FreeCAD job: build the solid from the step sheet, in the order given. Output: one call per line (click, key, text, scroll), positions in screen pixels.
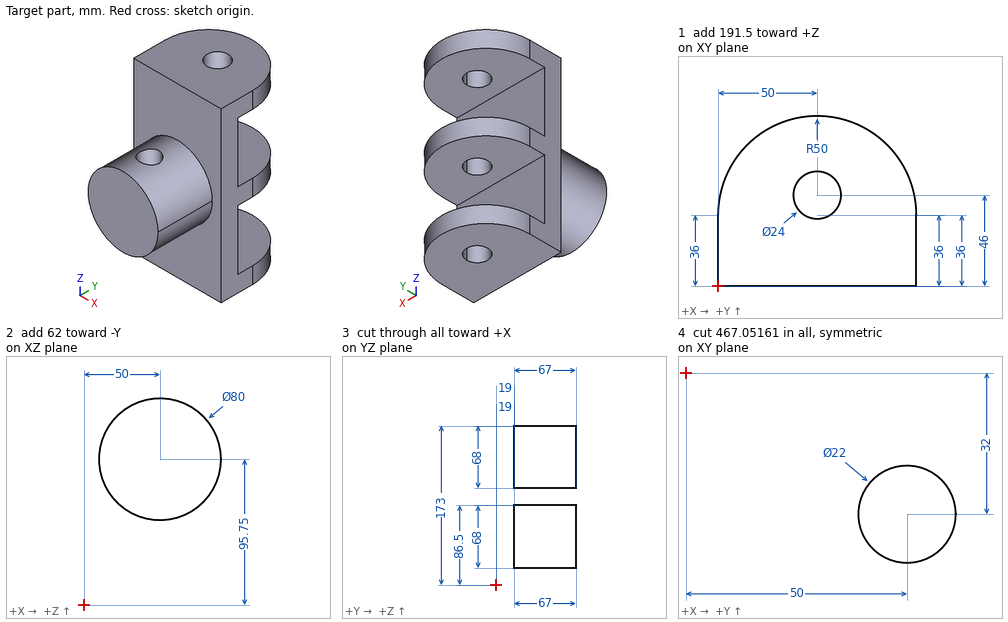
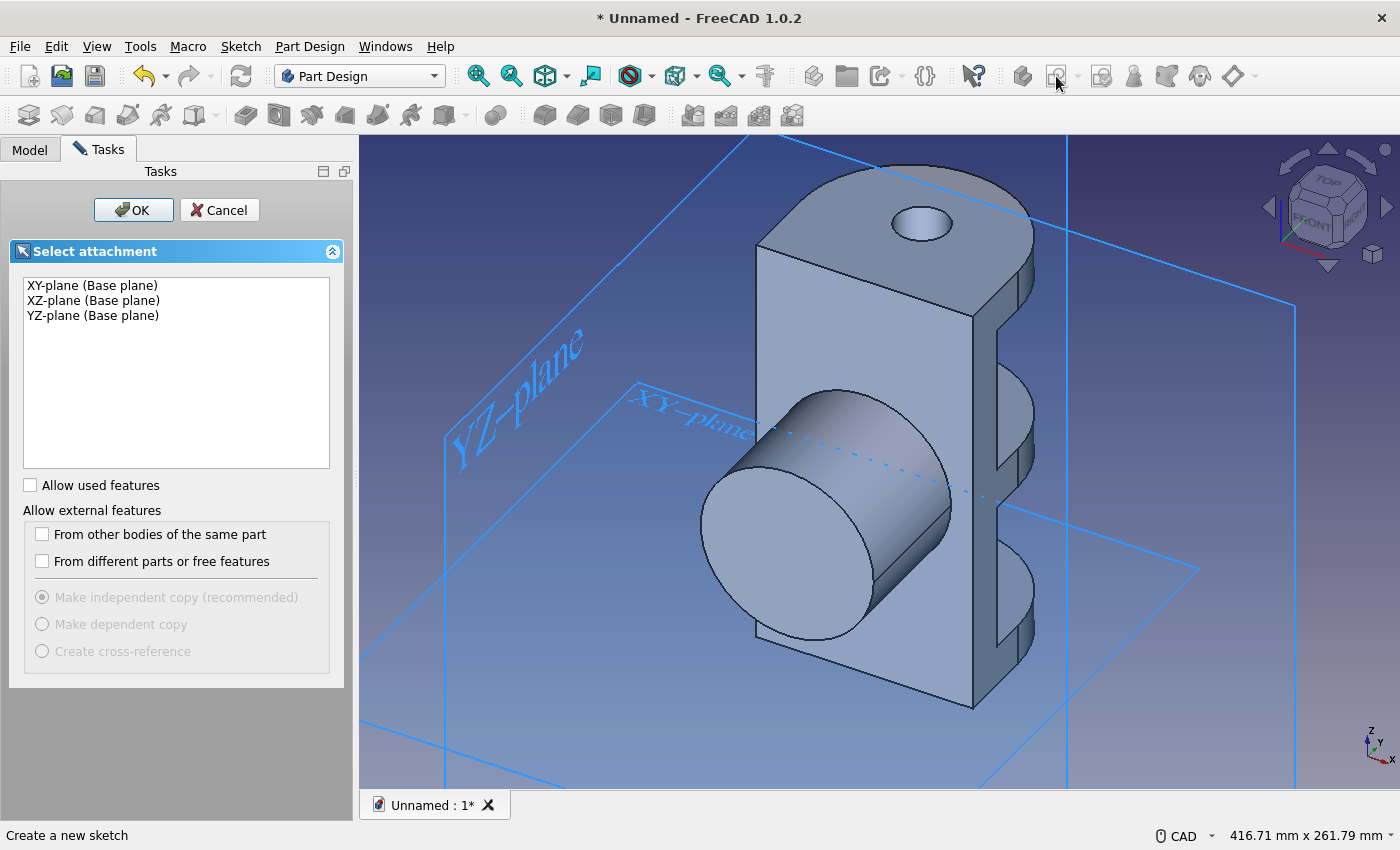
click(84, 286)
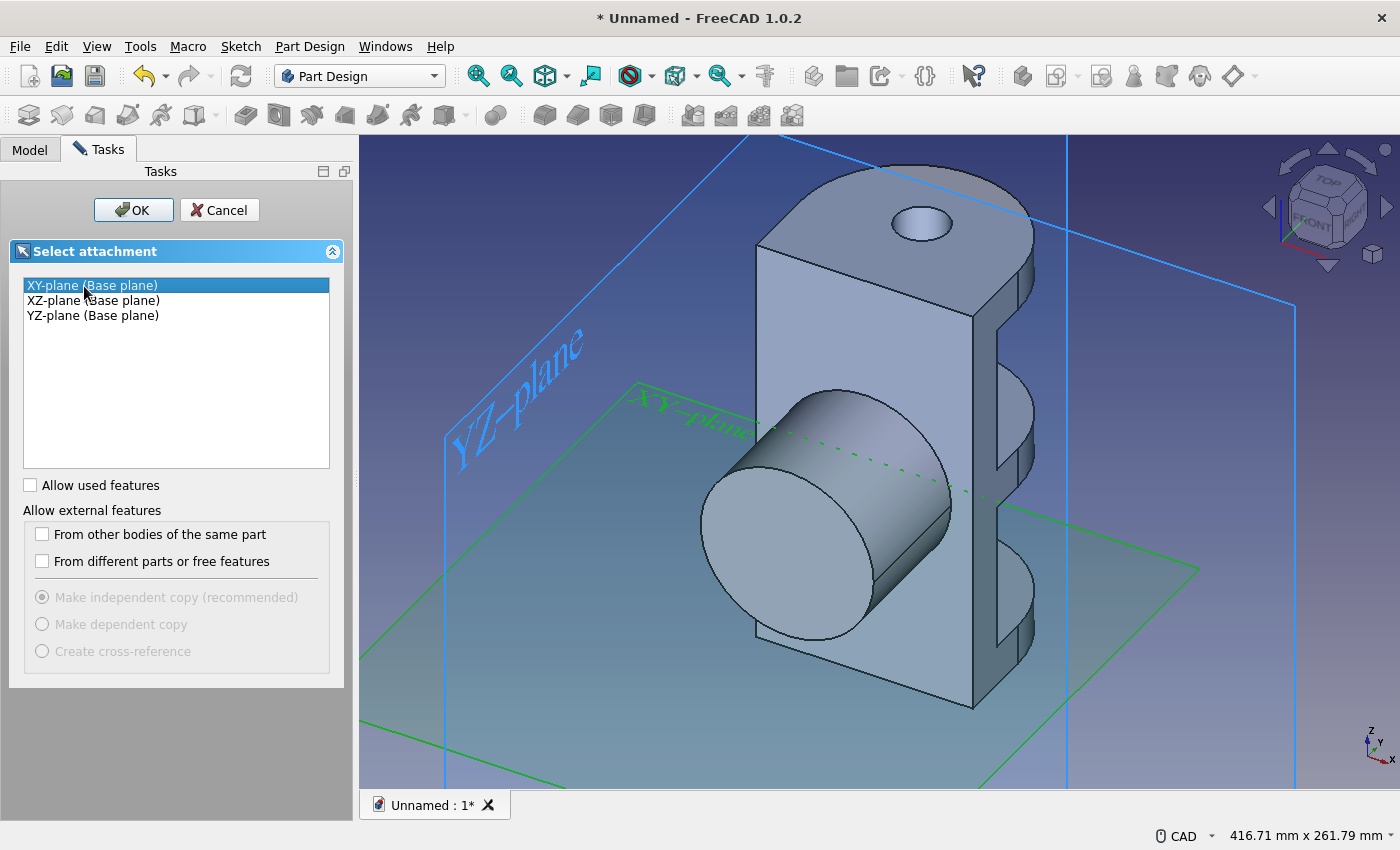
click(134, 210)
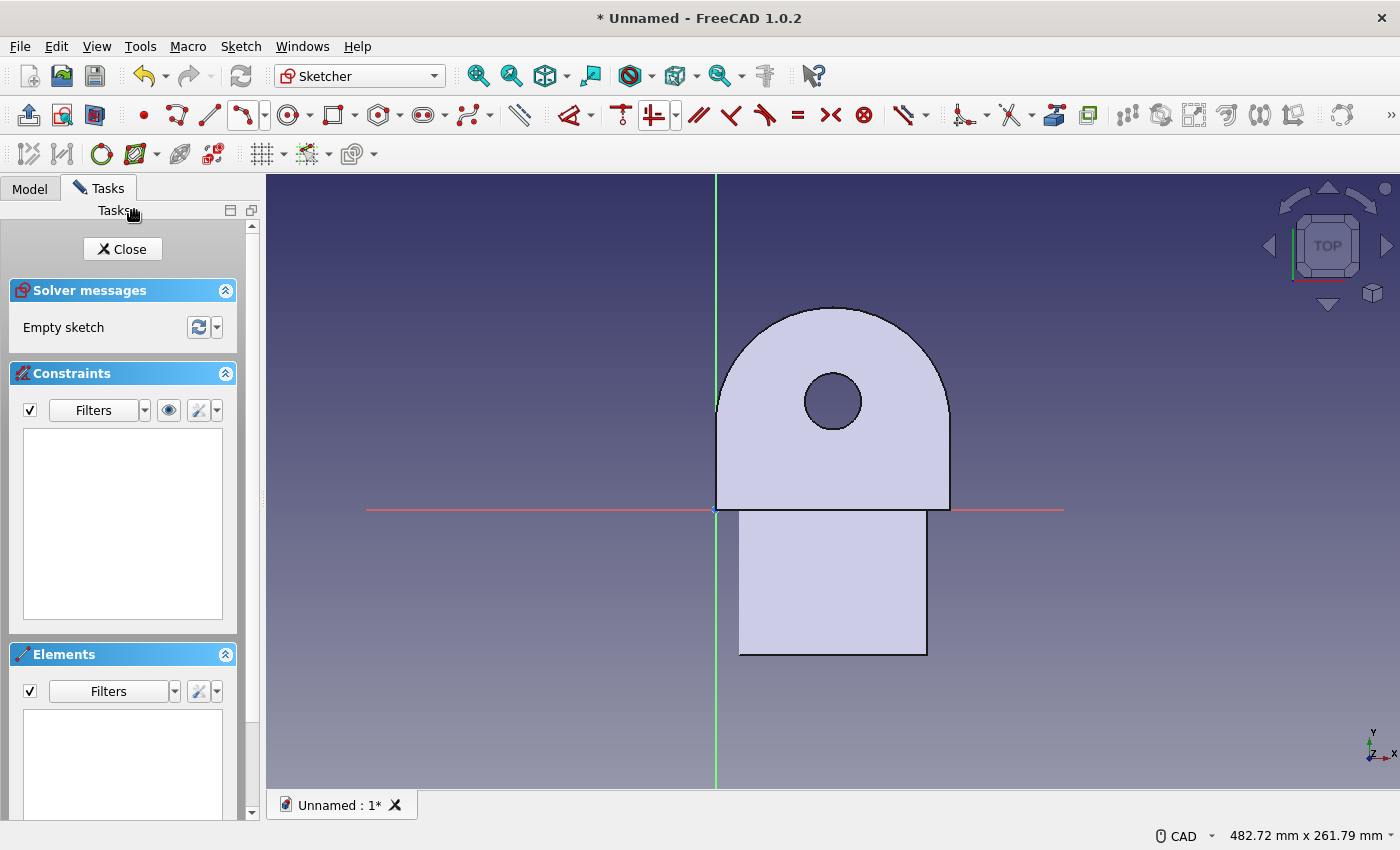
click(95, 116)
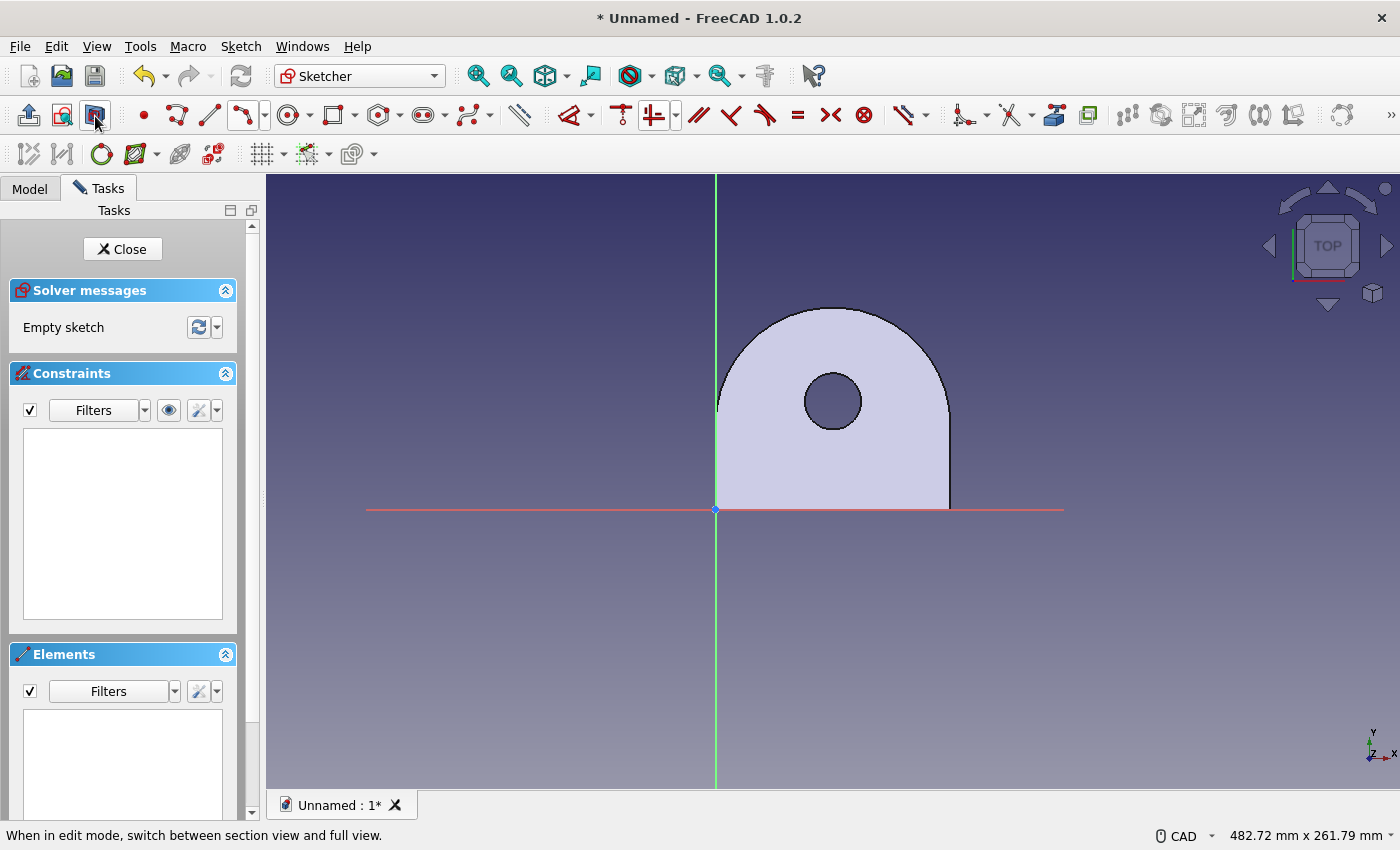
scroll(844, 601, up, 10)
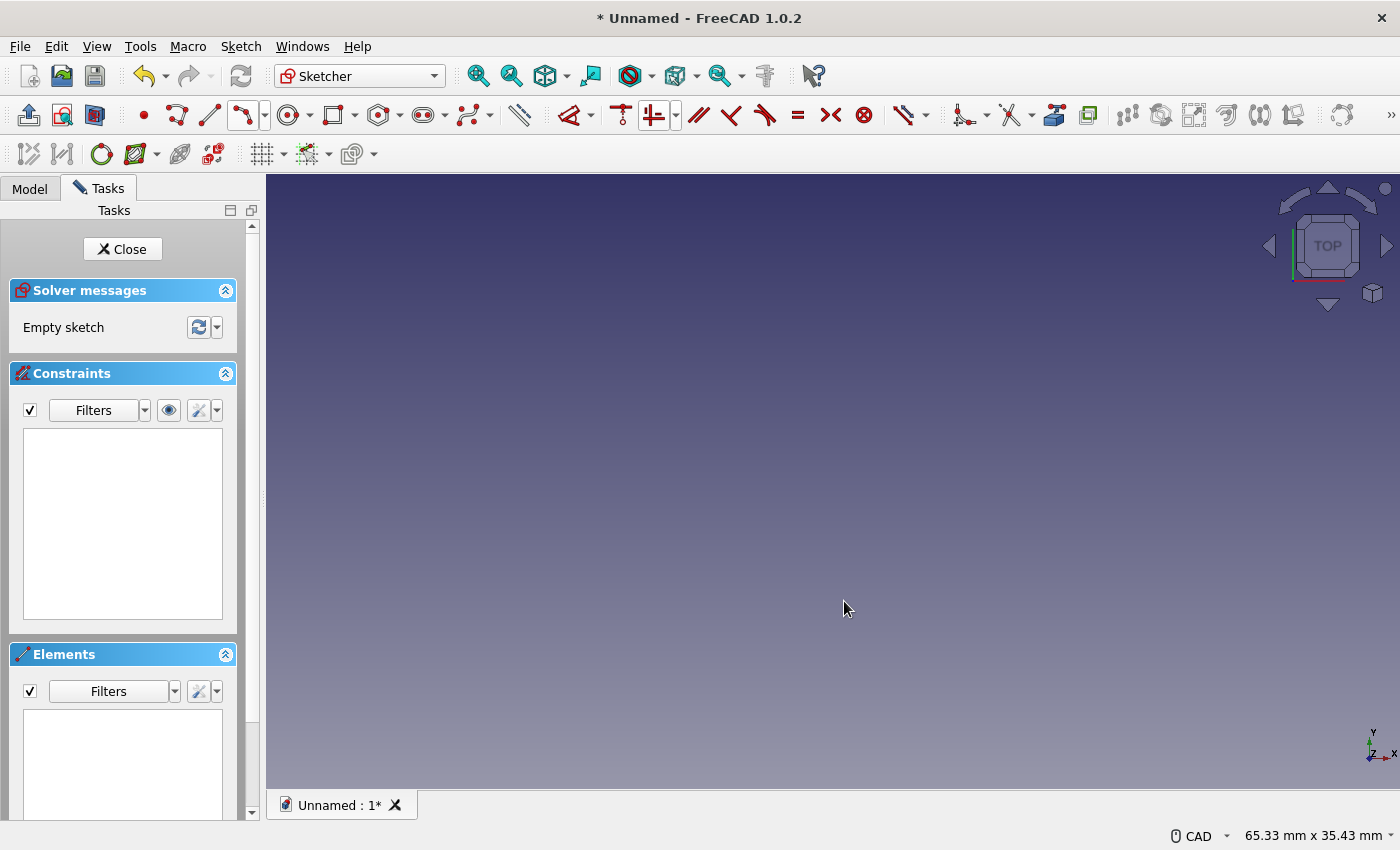
click(288, 116)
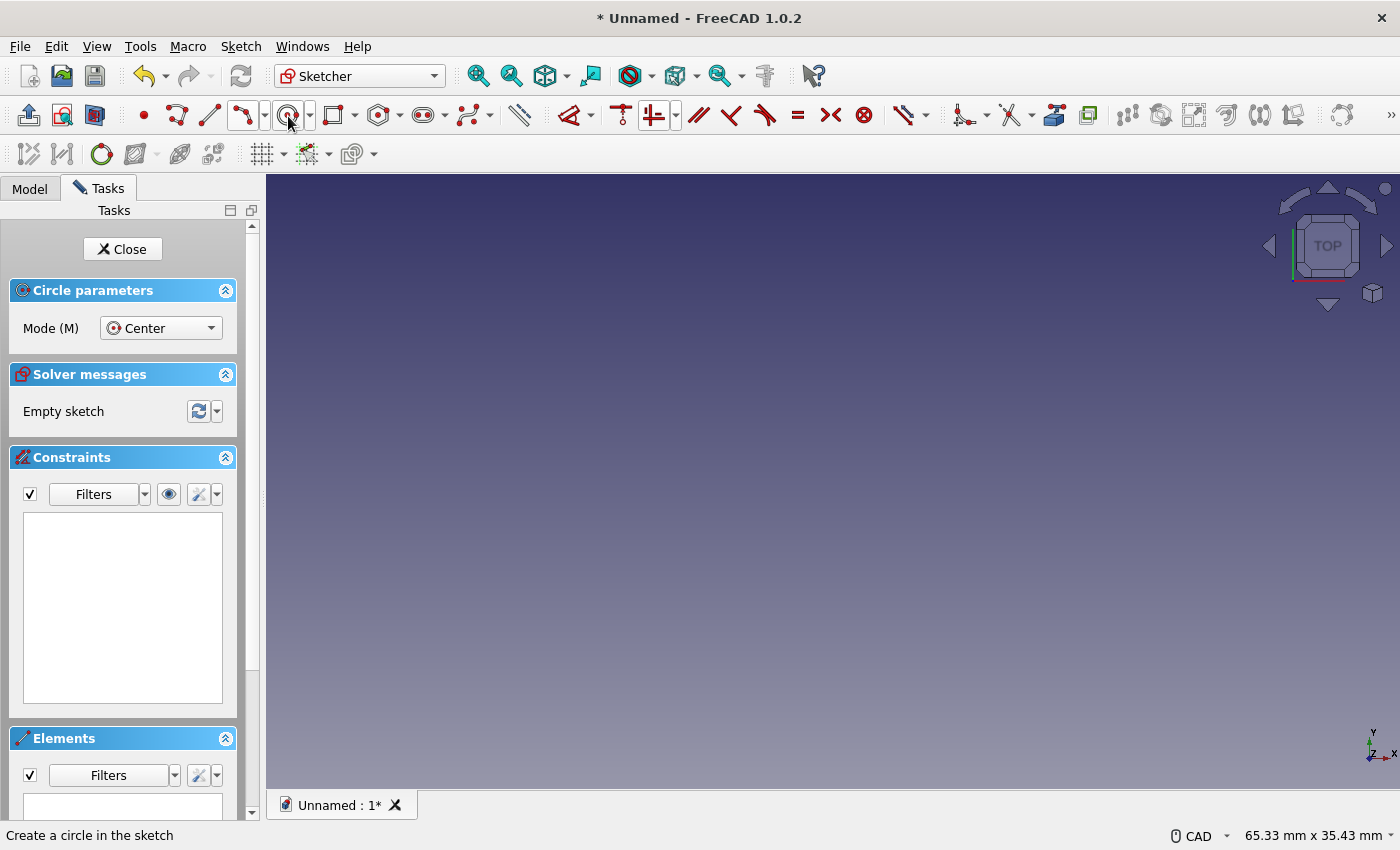
click(759, 476)
click(894, 341)
key(Escape)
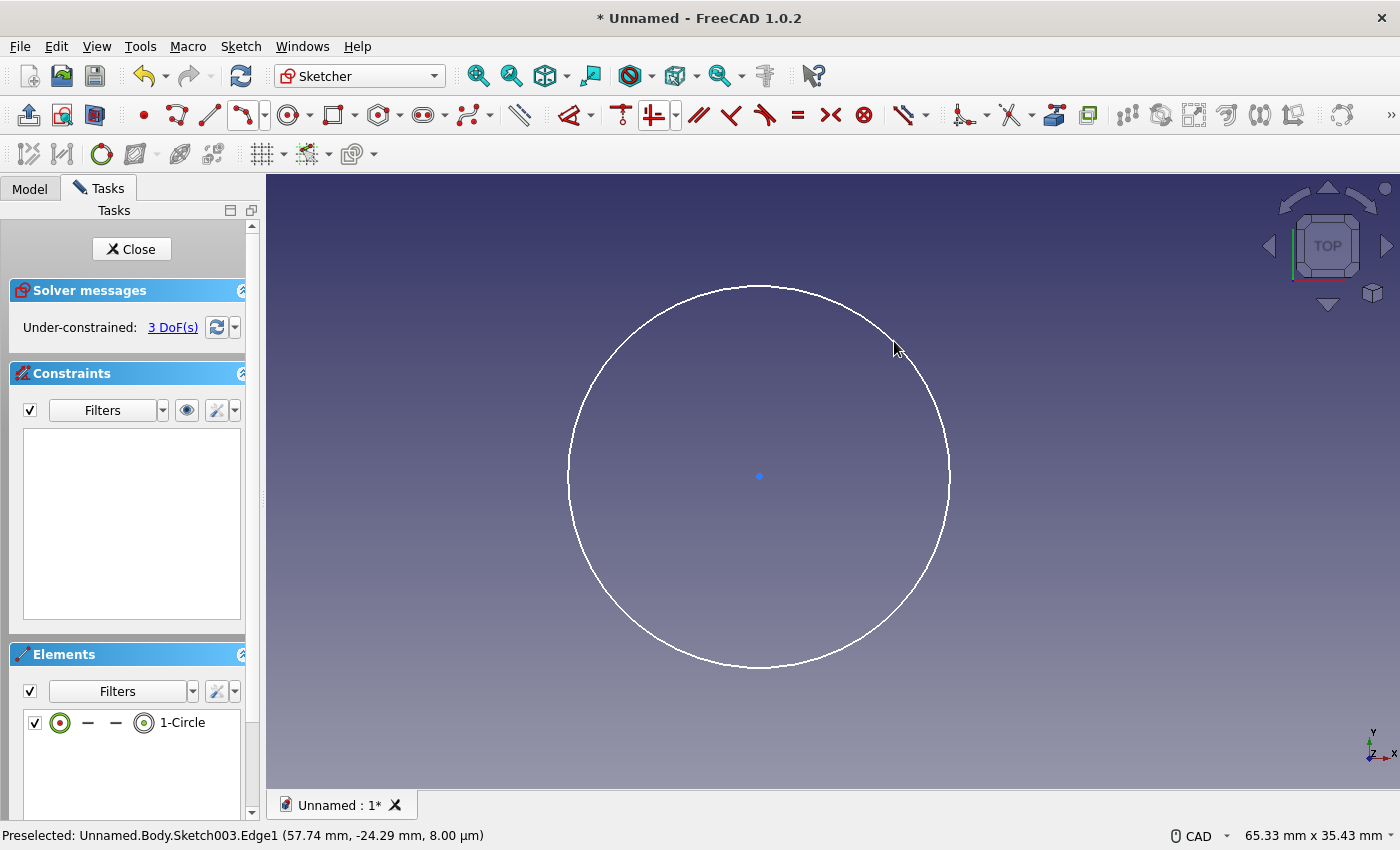
click(568, 116)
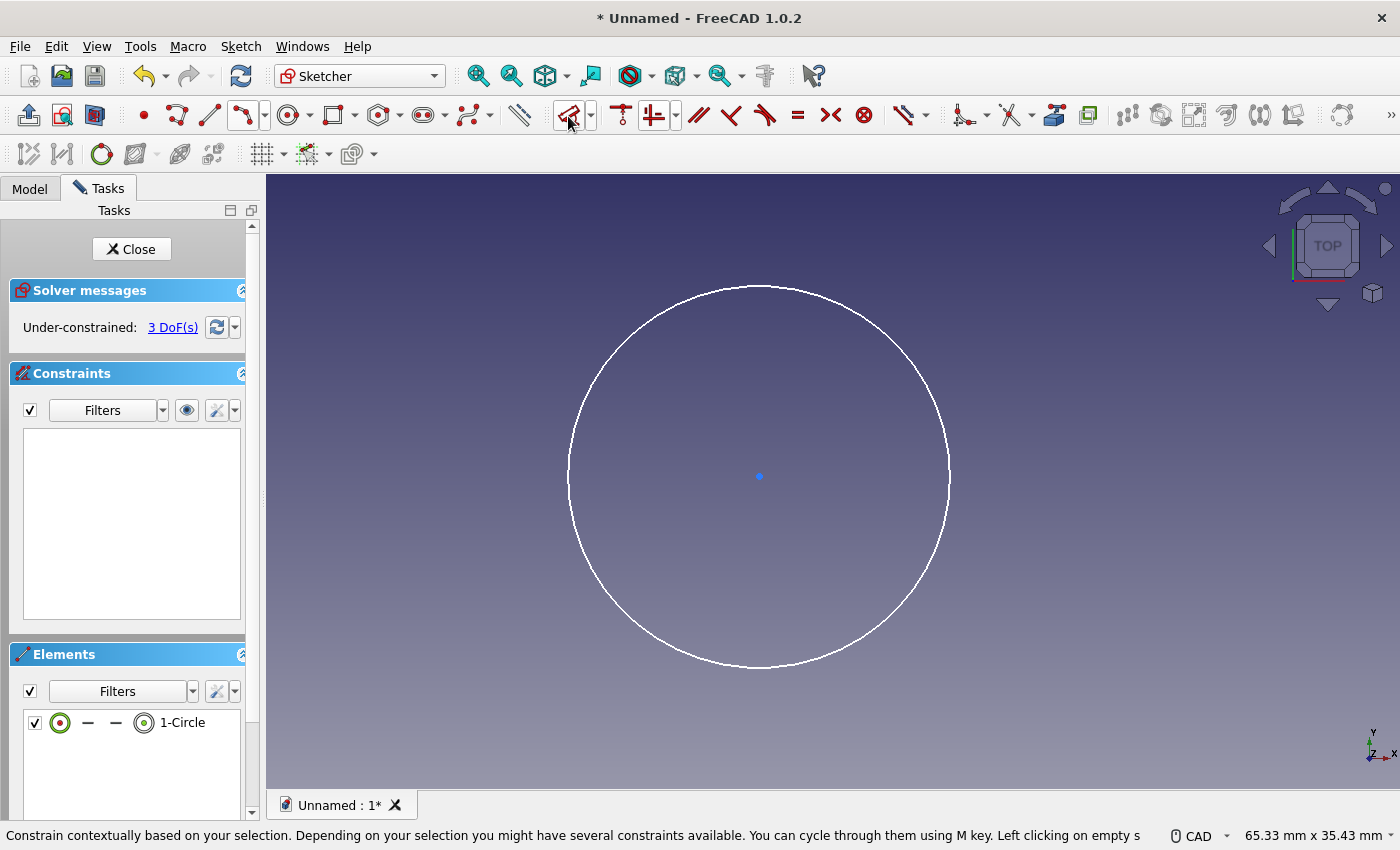
click(894, 342)
click(917, 319)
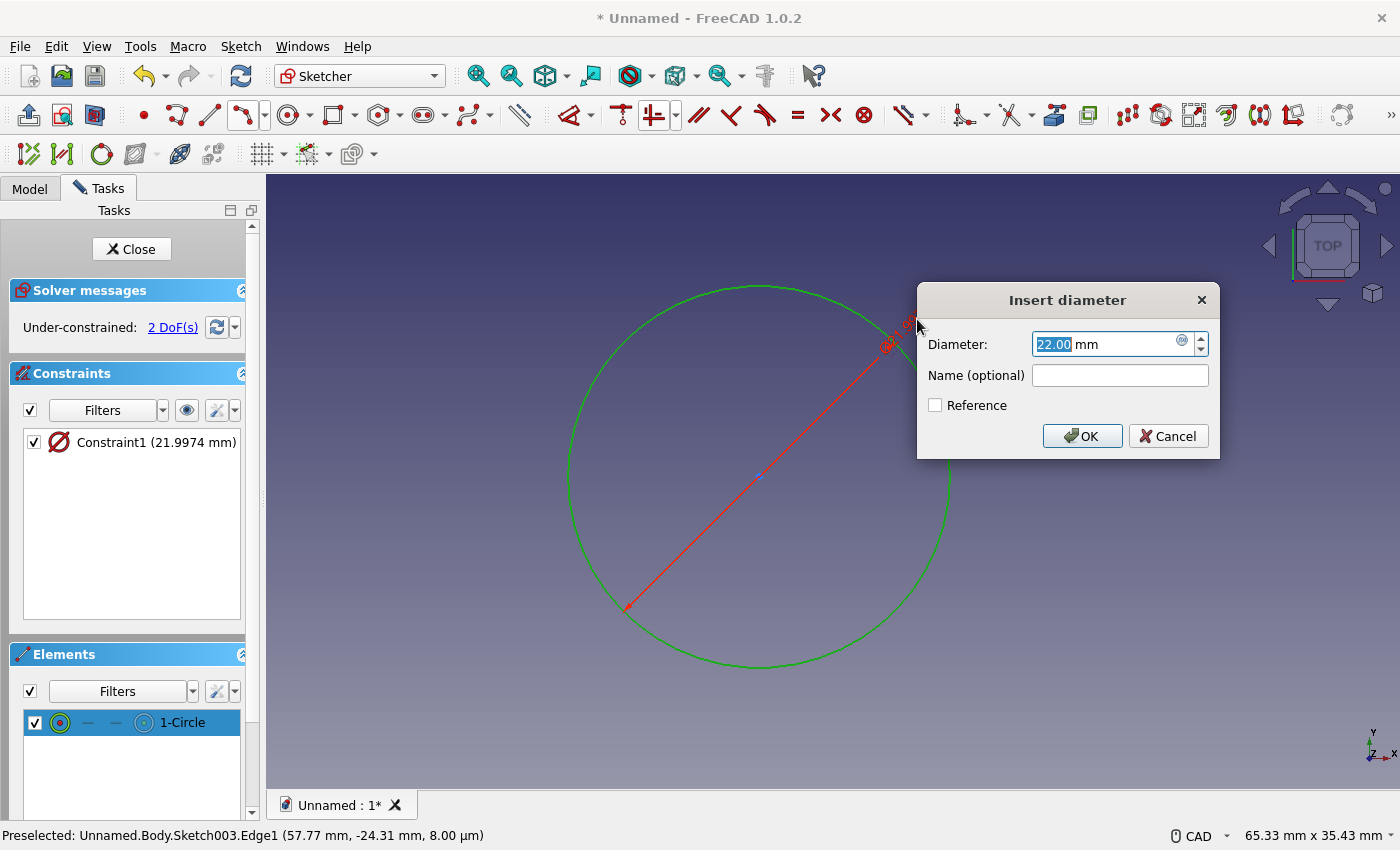
text(22)
key(Return)